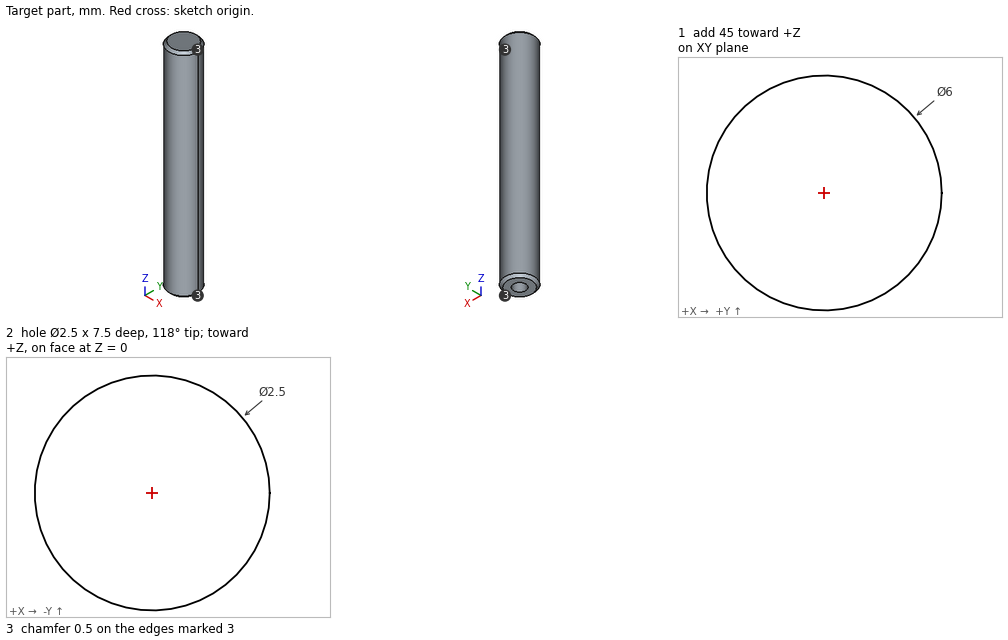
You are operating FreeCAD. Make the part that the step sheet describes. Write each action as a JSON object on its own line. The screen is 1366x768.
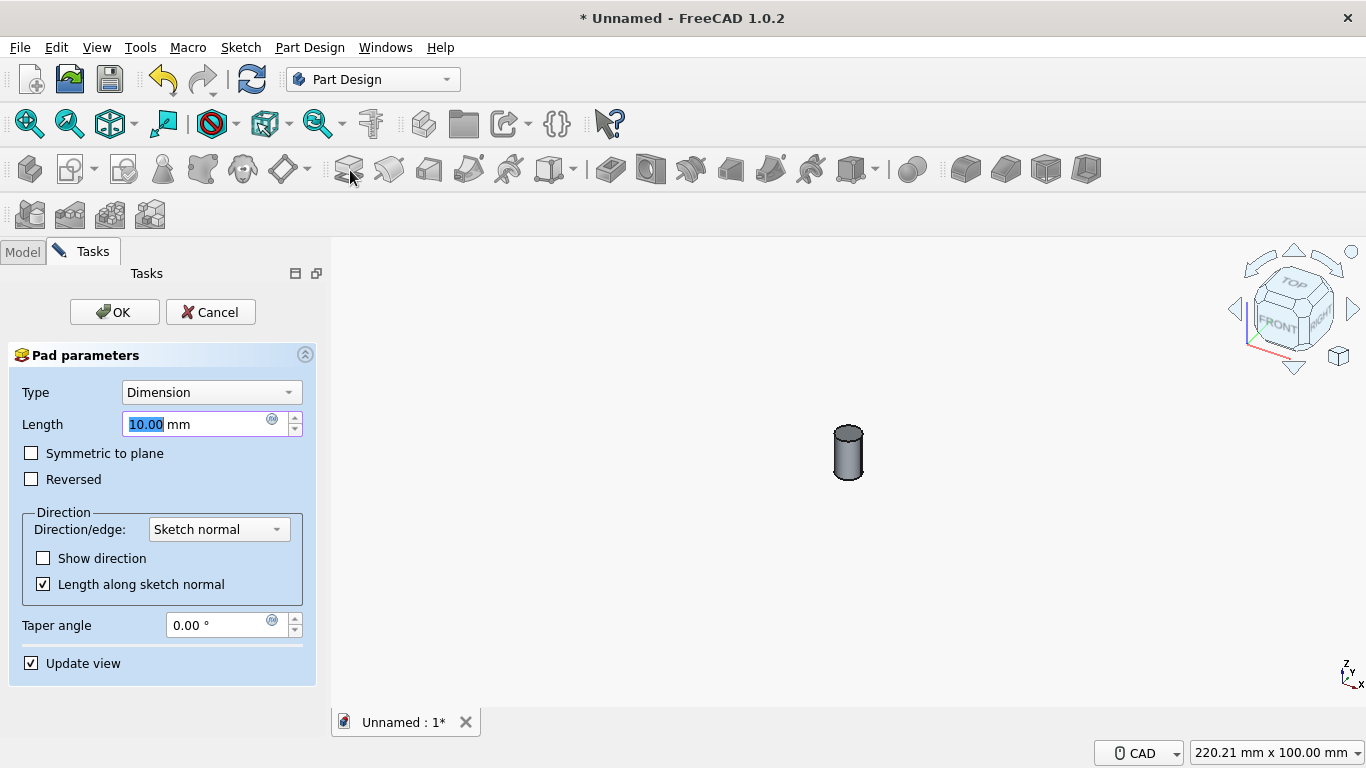
{"action": "type", "text": "45"}
{"action": "key", "text": "Tab"}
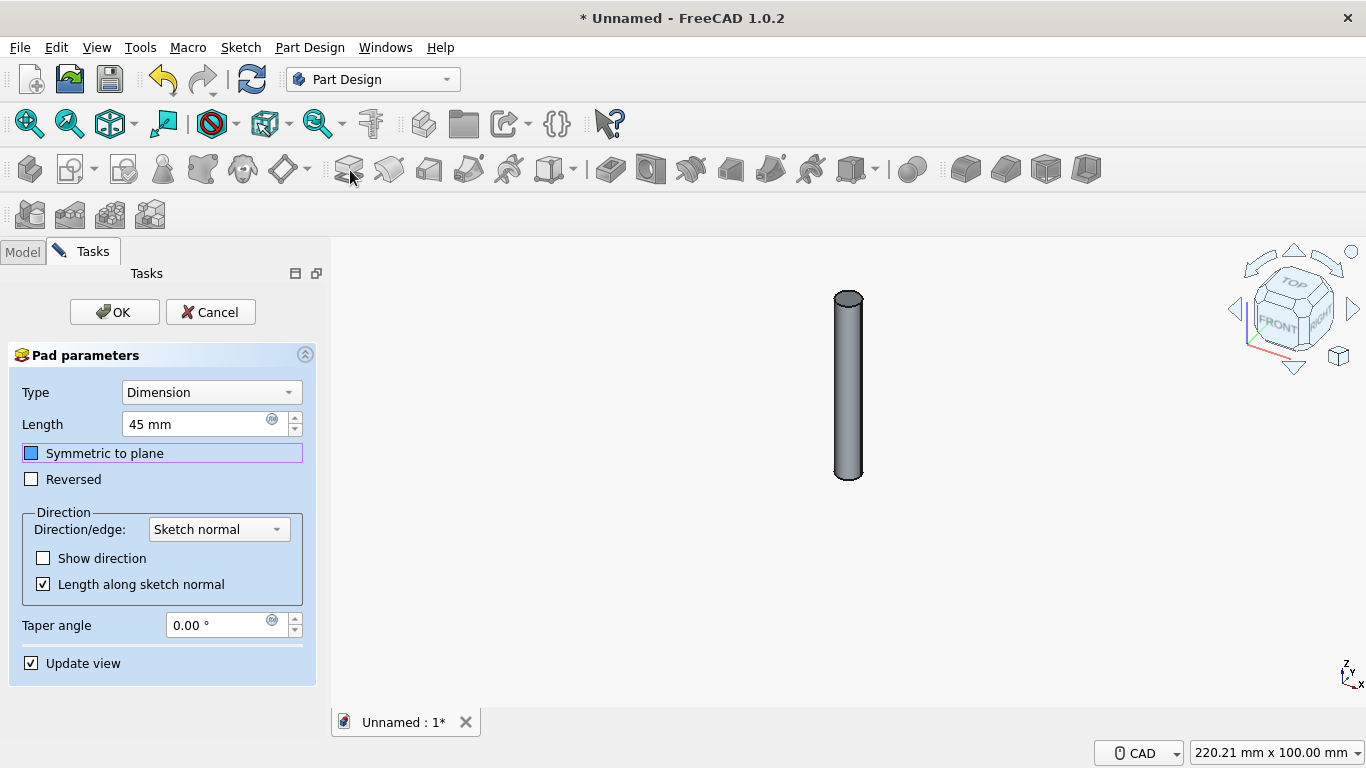
{"action": "left_click", "coordinate": [115, 312]}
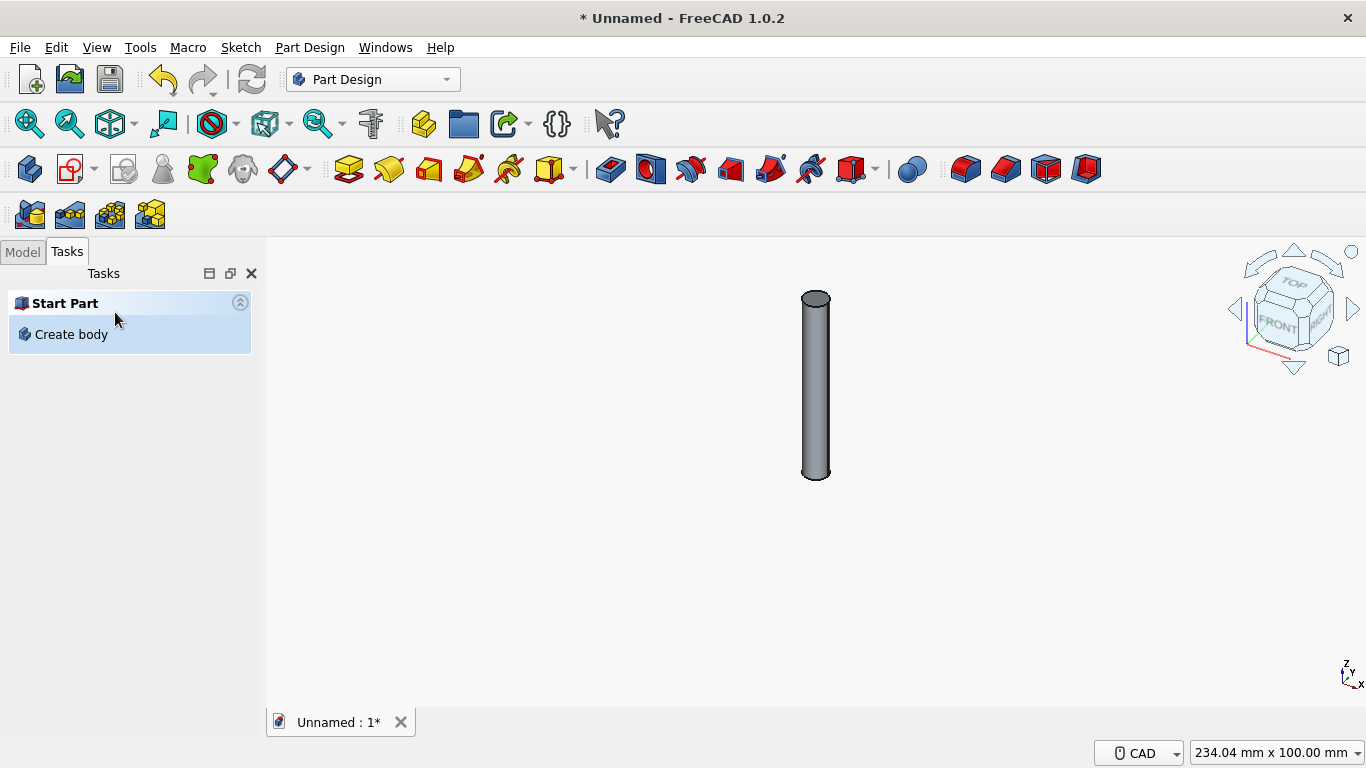
{"action": "left_click", "coordinate": [30, 124]}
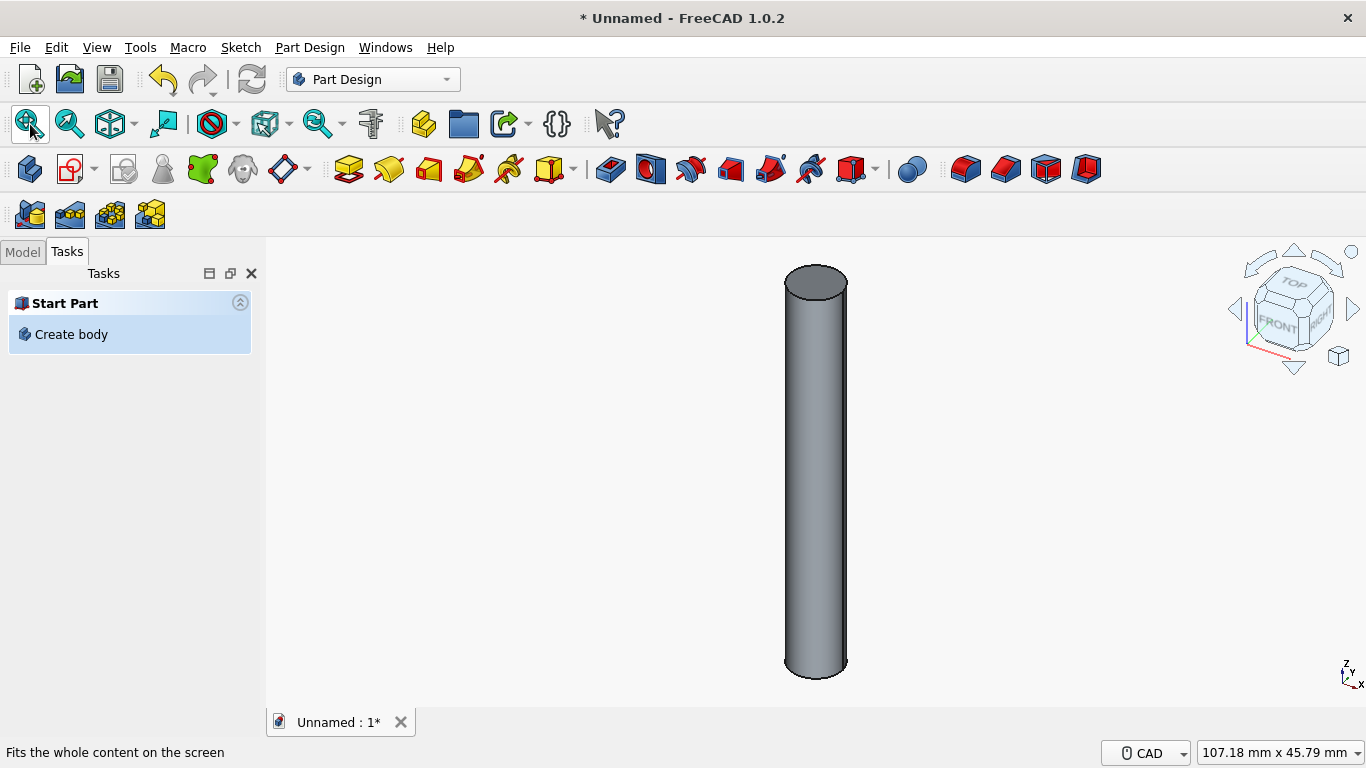
{"action": "key", "text": "5"}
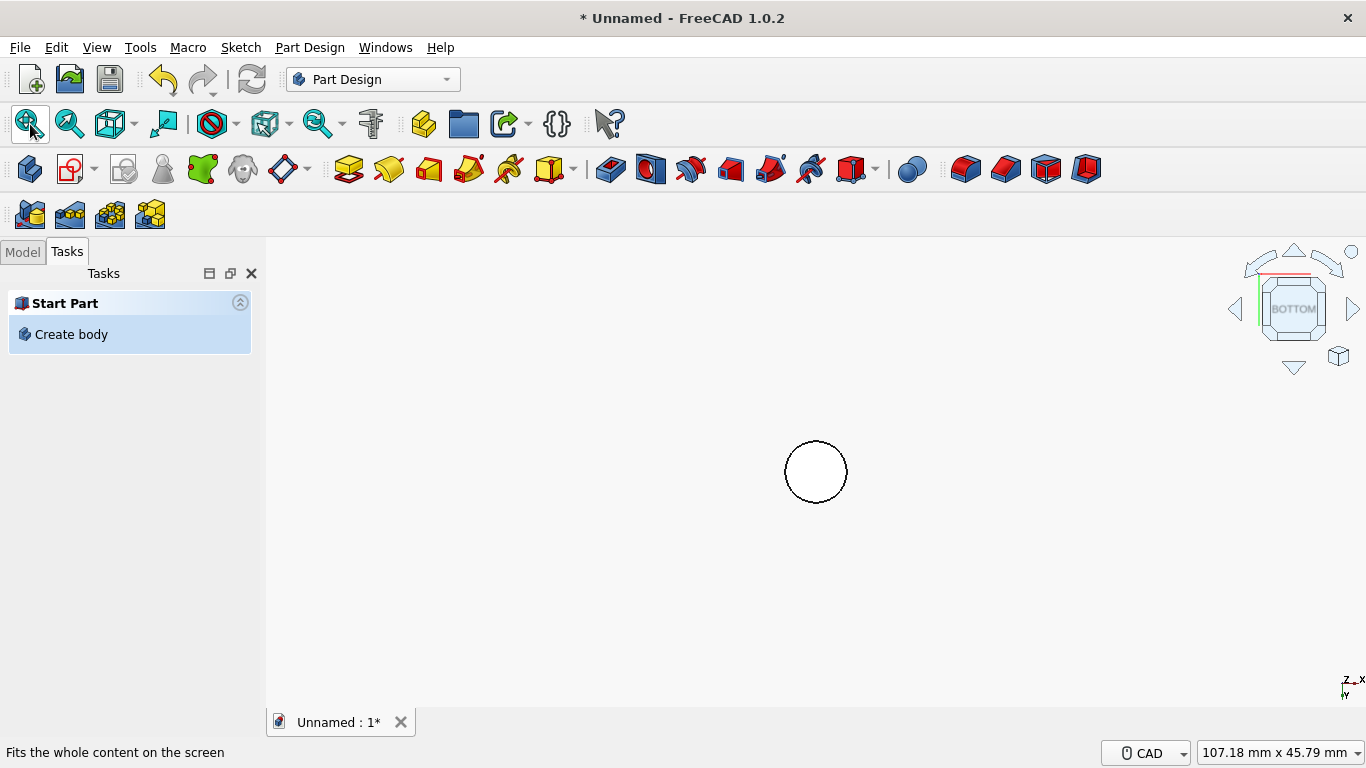
{"action": "left_click", "coordinate": [30, 124]}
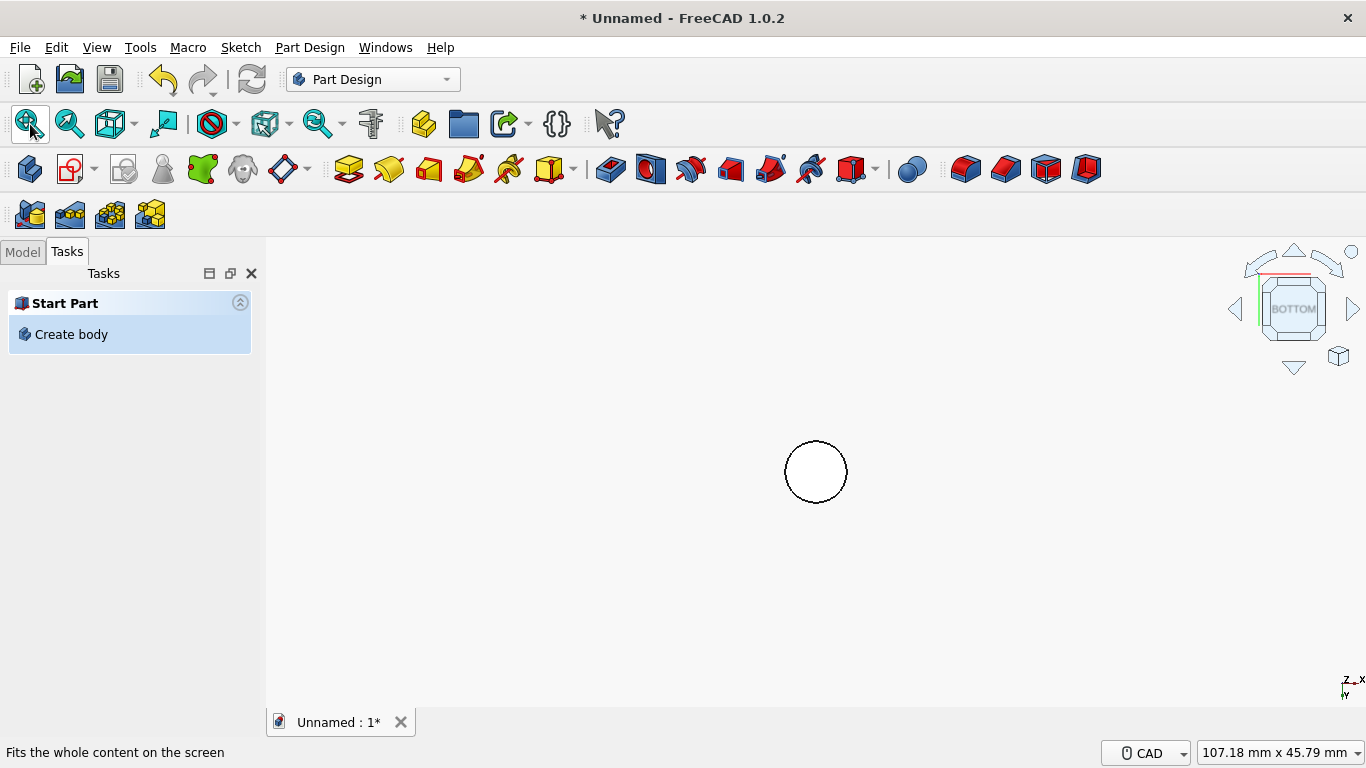
{"action": "left_click", "coordinate": [816, 471]}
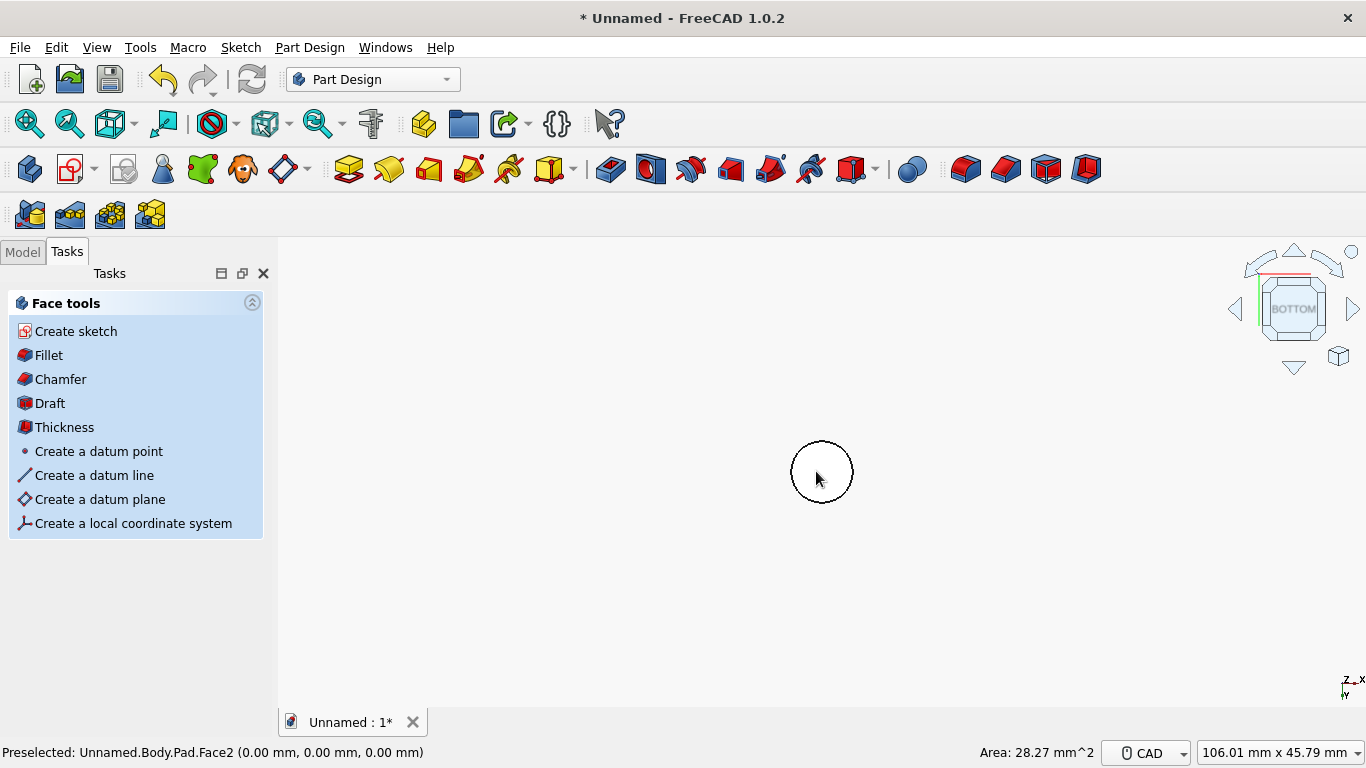
{"action": "left_click", "coordinate": [70, 170]}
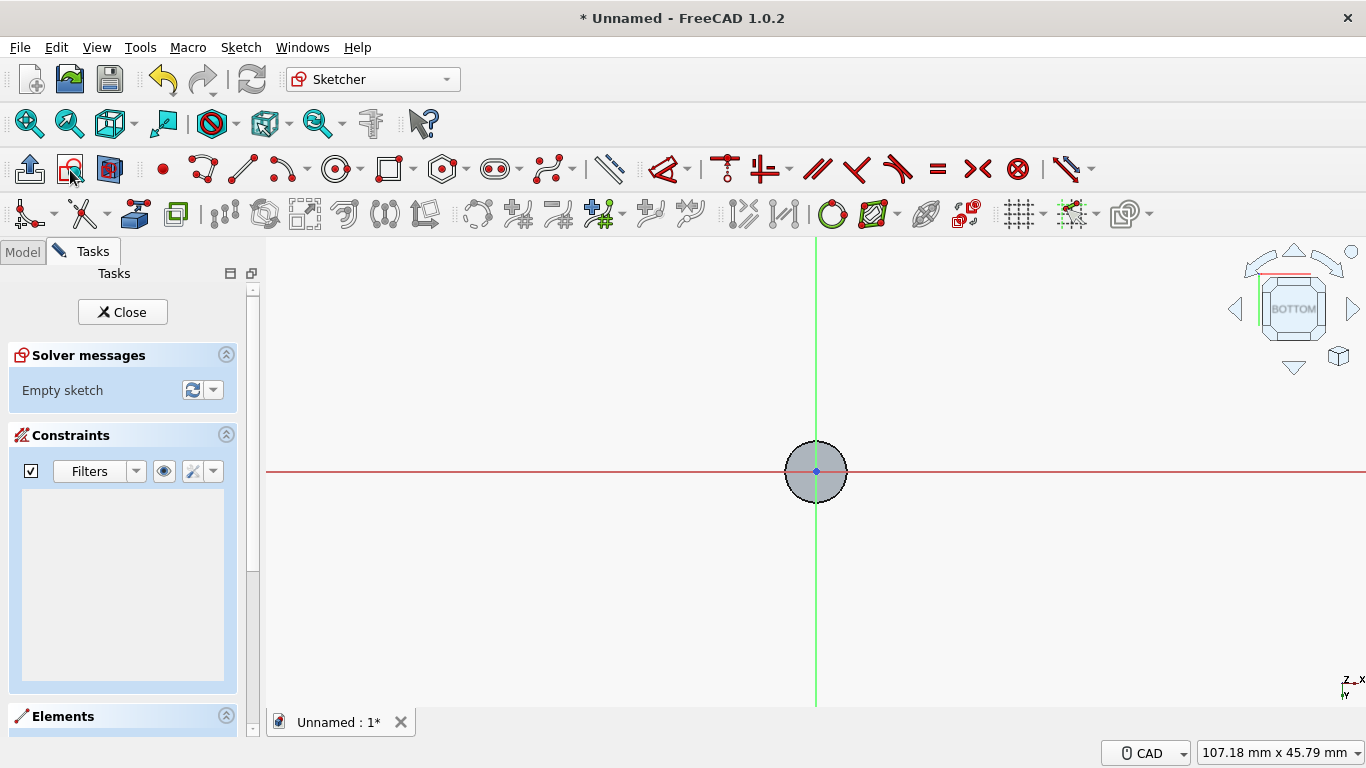
{"action": "scroll", "coordinate": [823, 472], "scroll_direction": "up", "scroll_amount": 12}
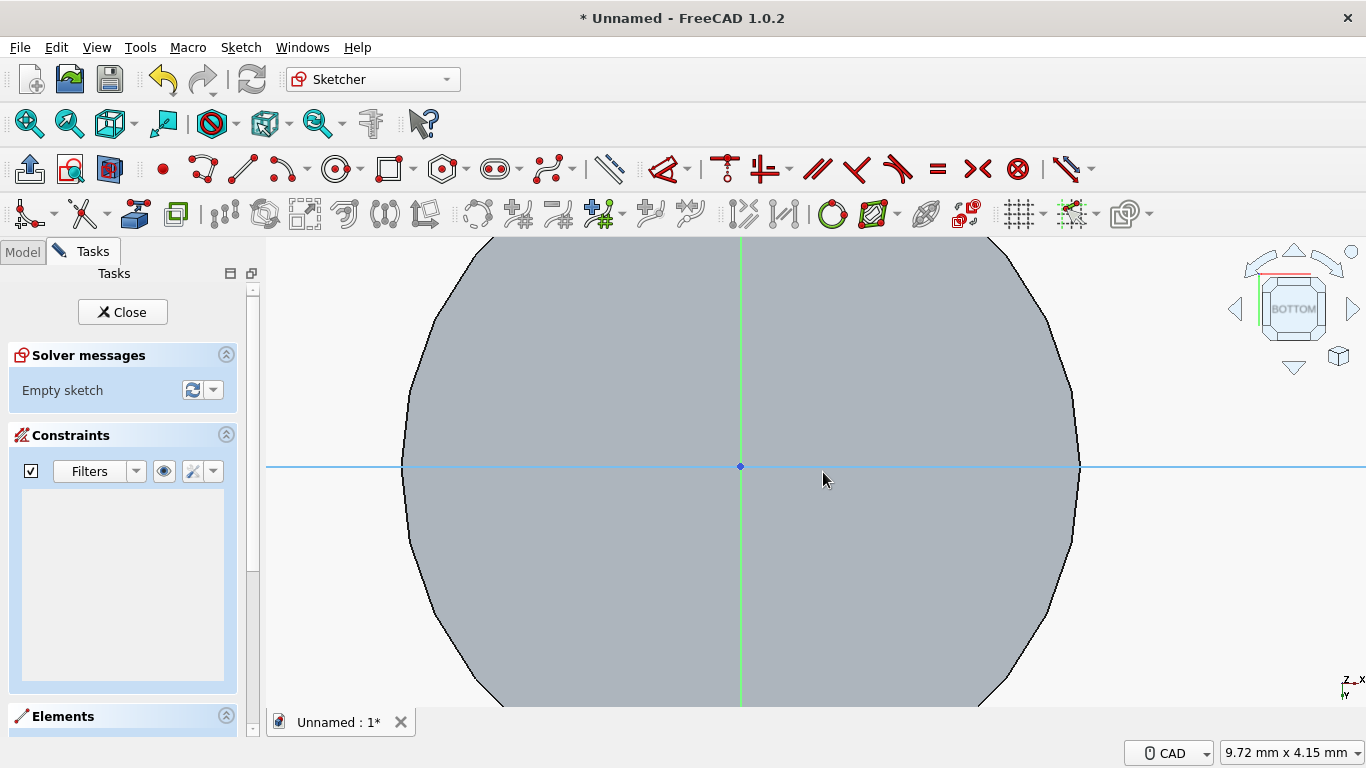
{"action": "left_click", "coordinate": [336, 170]}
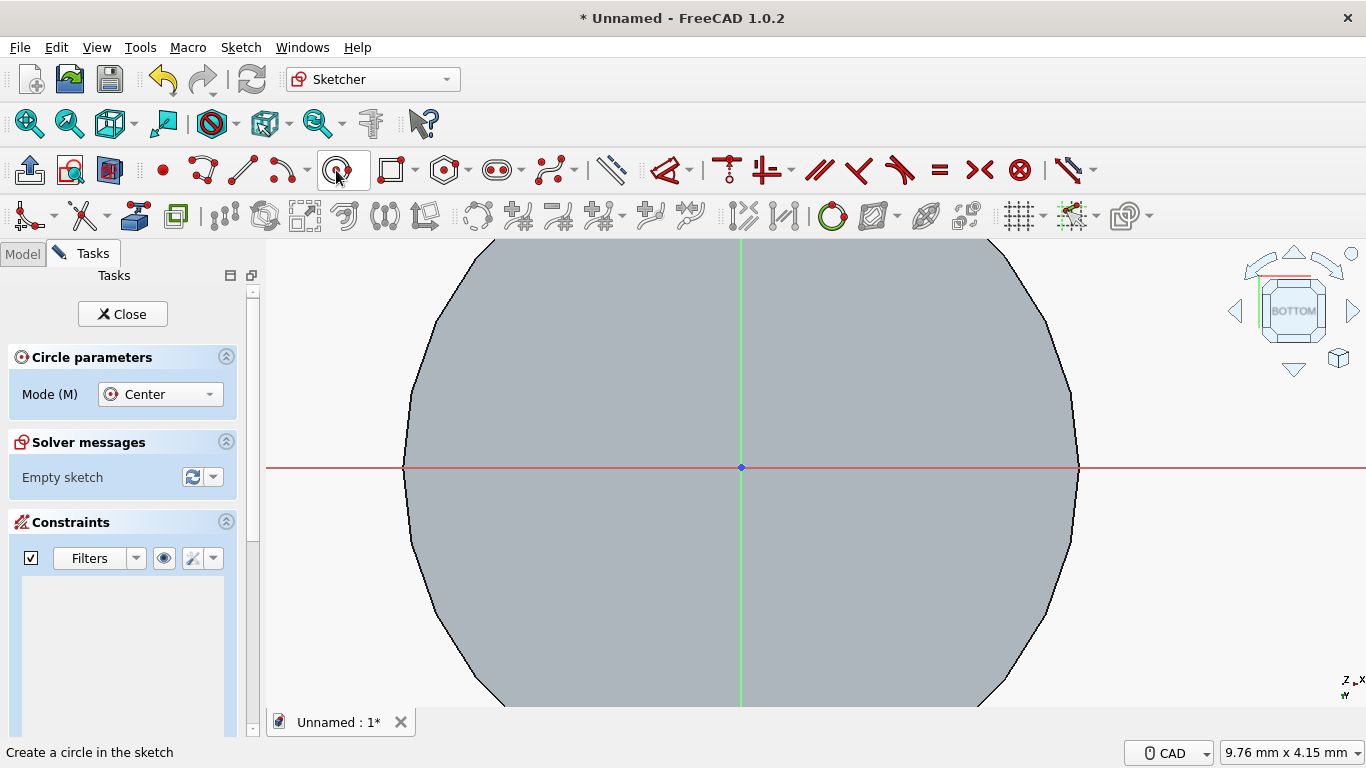
{"action": "left_click", "coordinate": [741, 468]}
{"action": "mouse_move", "coordinate": [841, 368]}